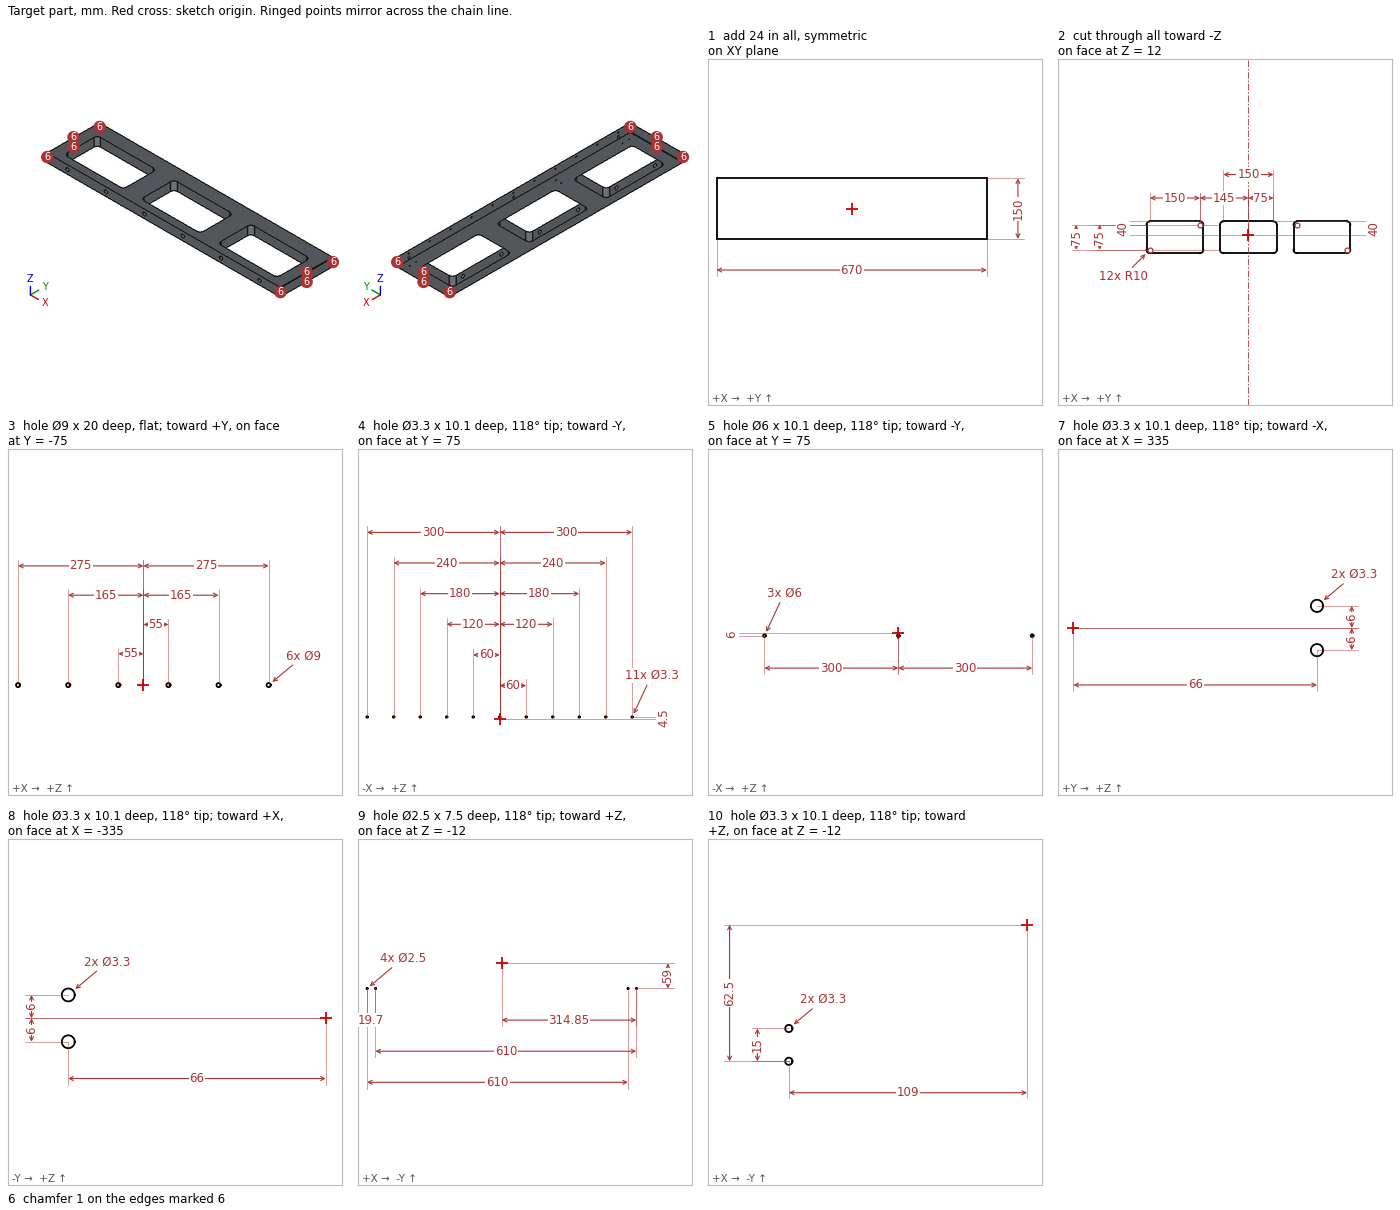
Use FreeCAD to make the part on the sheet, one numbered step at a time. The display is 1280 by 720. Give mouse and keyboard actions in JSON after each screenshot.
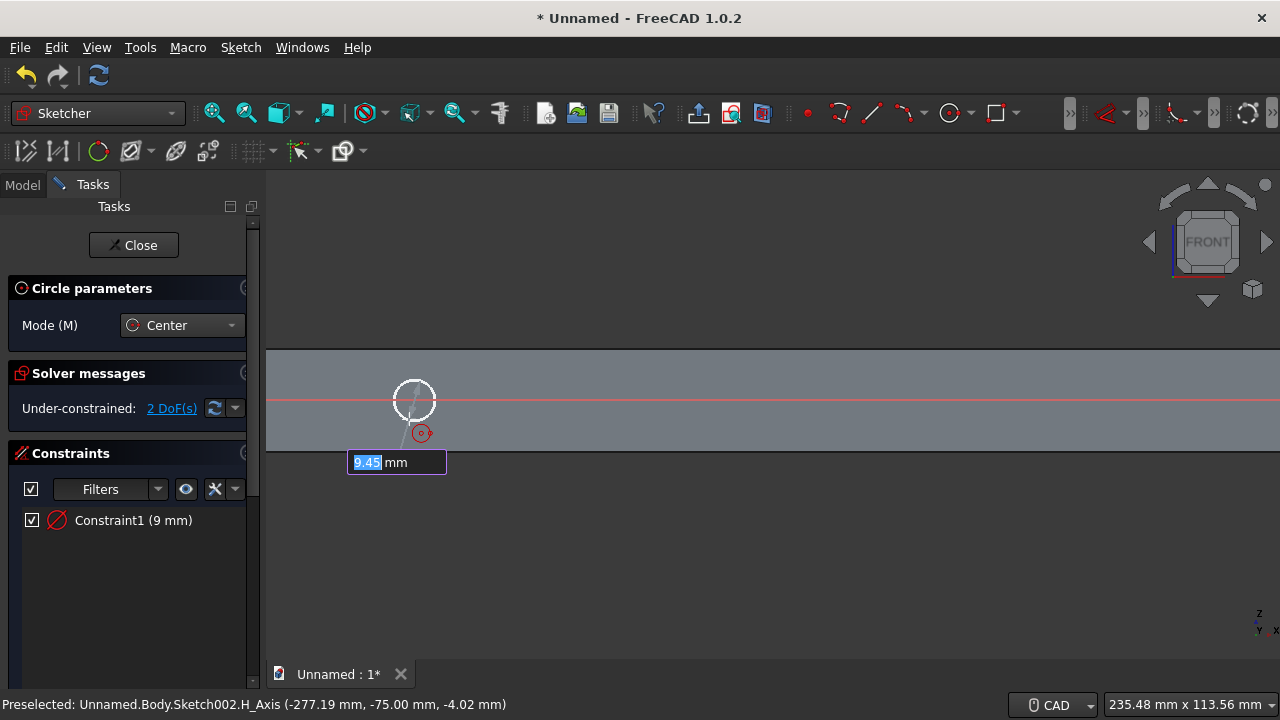
{"action": "type", "text": "9"}
{"action": "key", "text": "Return"}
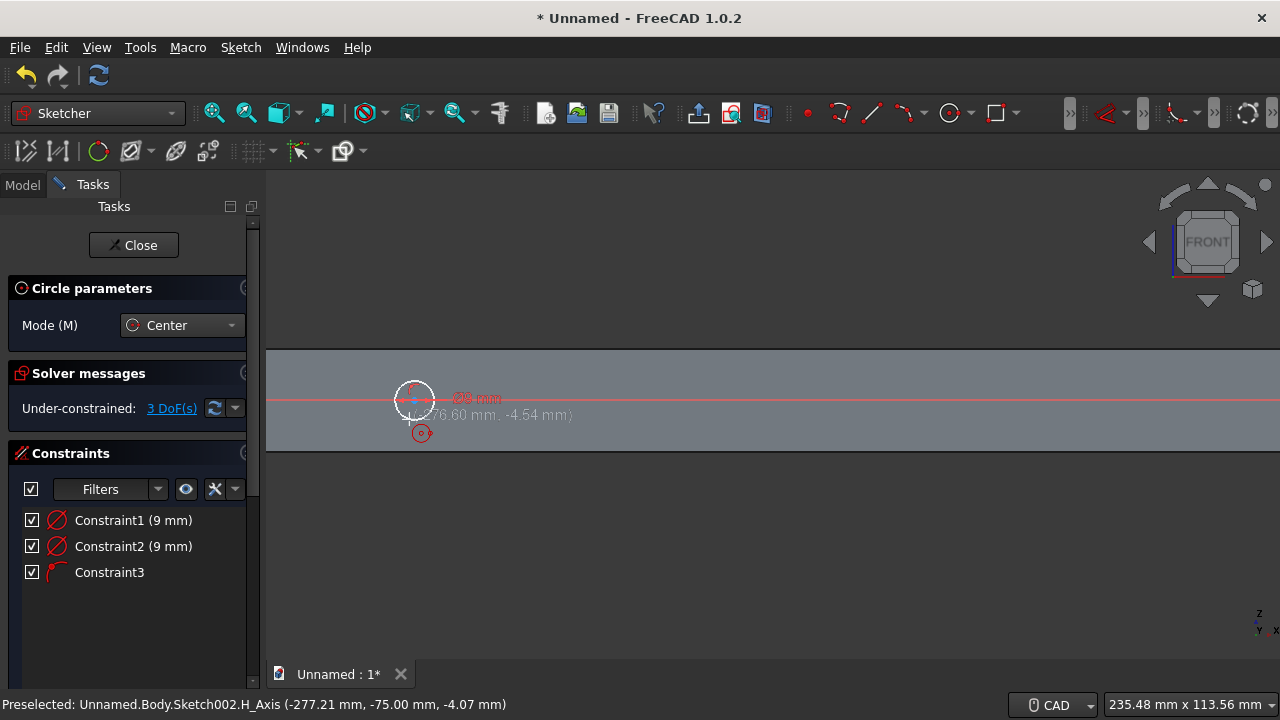
{"action": "scroll", "coordinate": [411, 419], "scroll_direction": "down", "scroll_amount": 7}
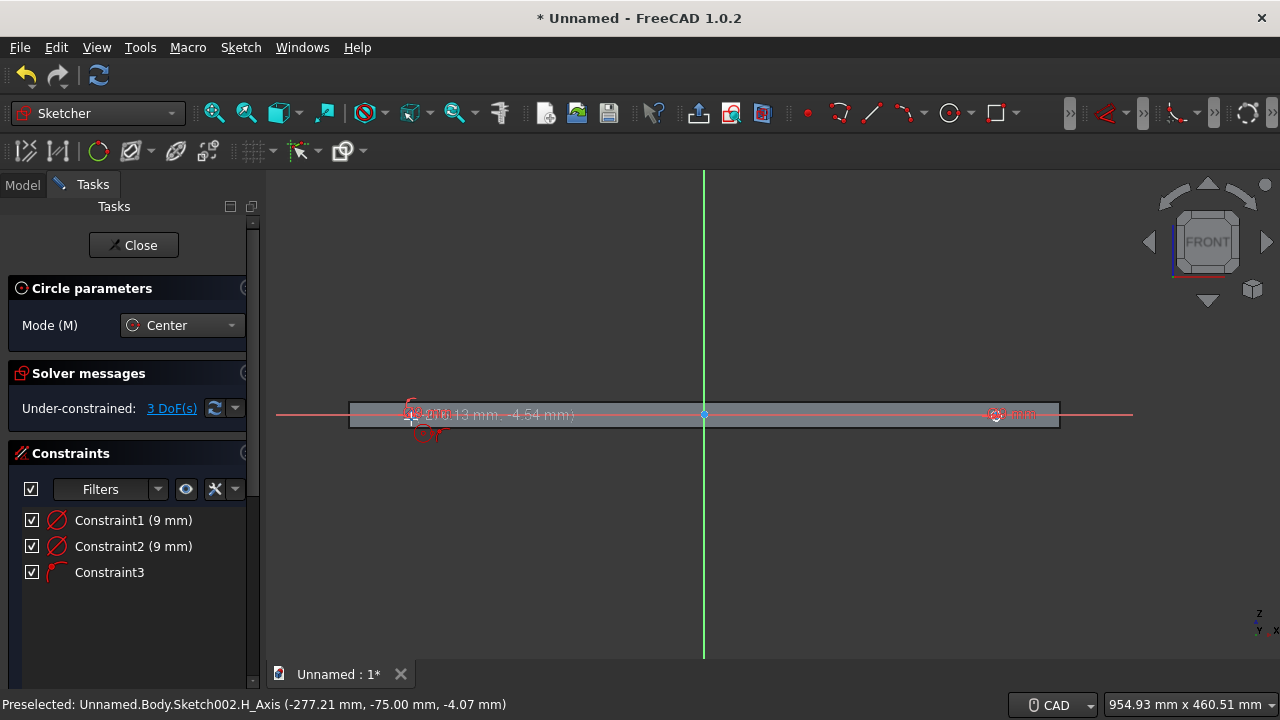
{"action": "left_click", "coordinate": [529, 415]}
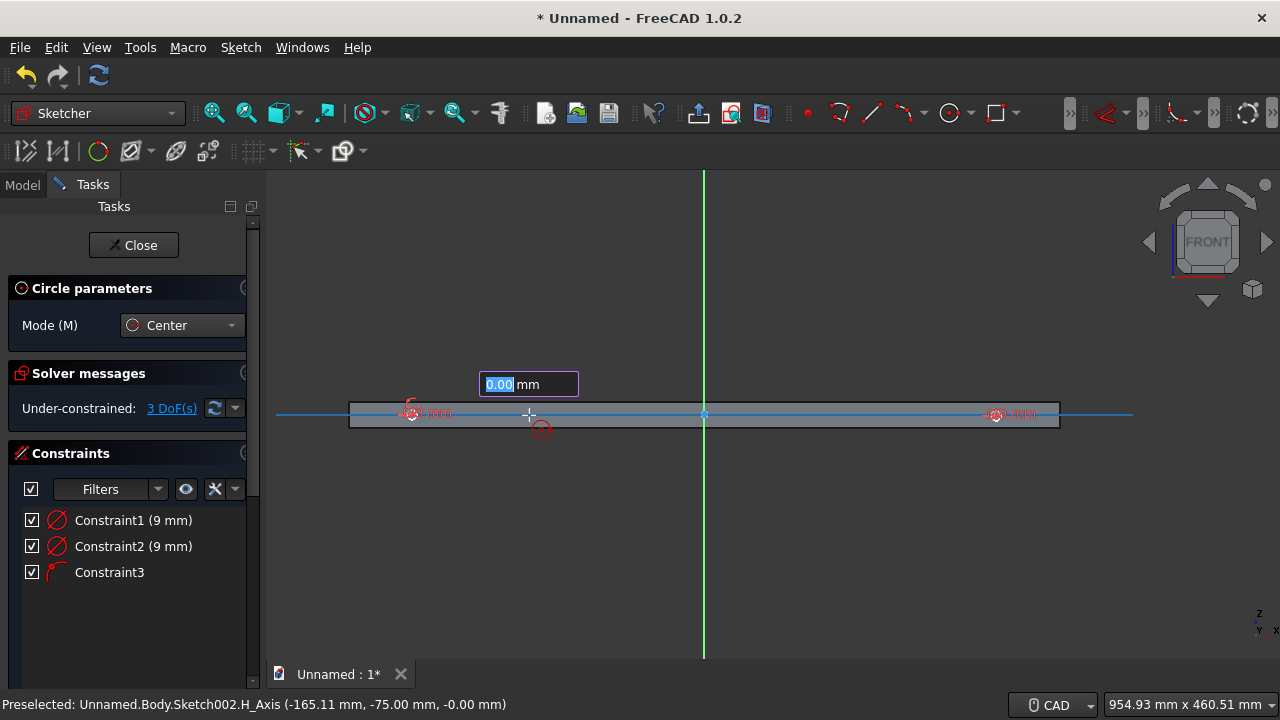
{"action": "scroll", "coordinate": [527, 419], "scroll_direction": "up", "scroll_amount": 7}
{"action": "mouse_move", "coordinate": [528, 419]}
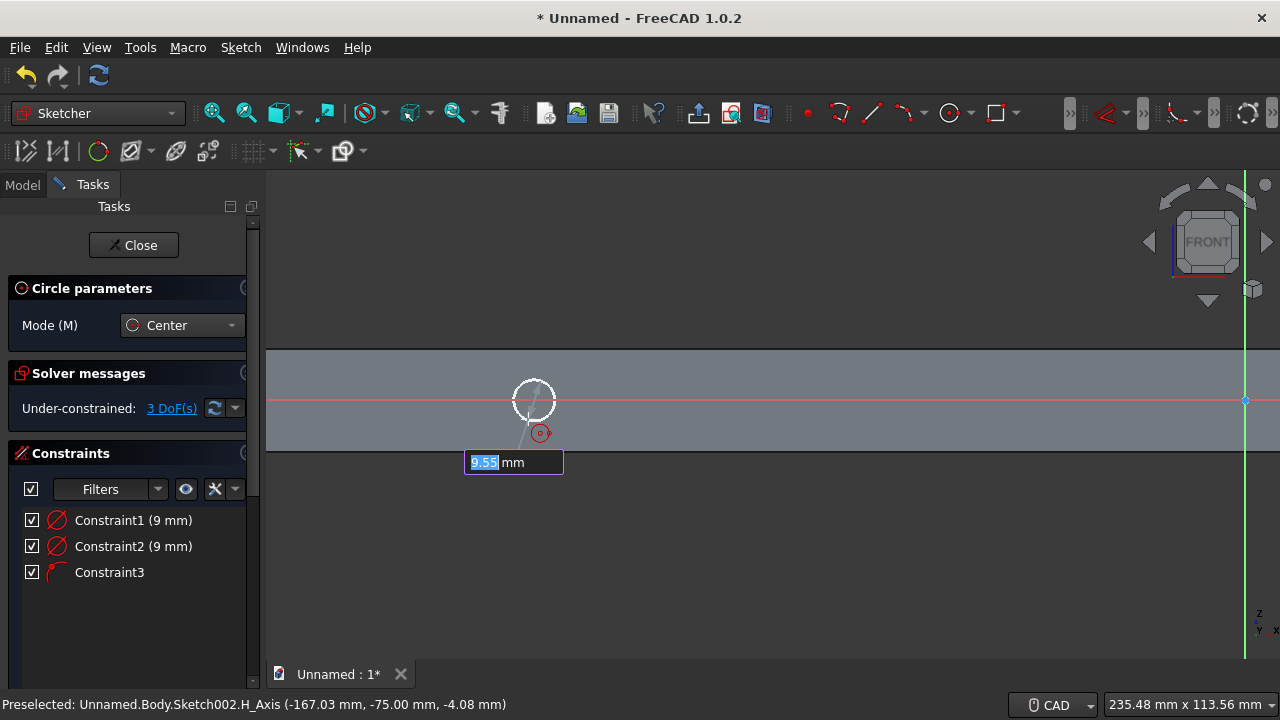
{"action": "type", "text": "9"}
{"action": "key", "text": "Return"}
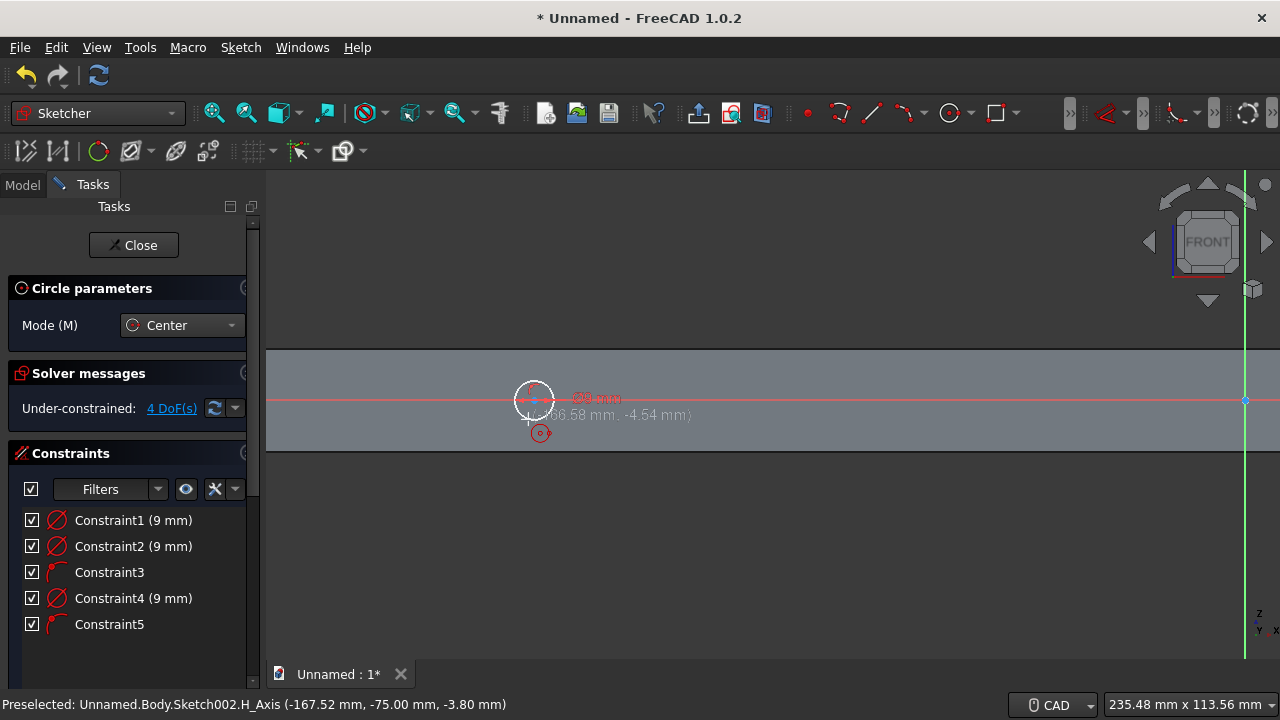
{"action": "scroll", "coordinate": [527, 419], "scroll_direction": "down", "scroll_amount": 7}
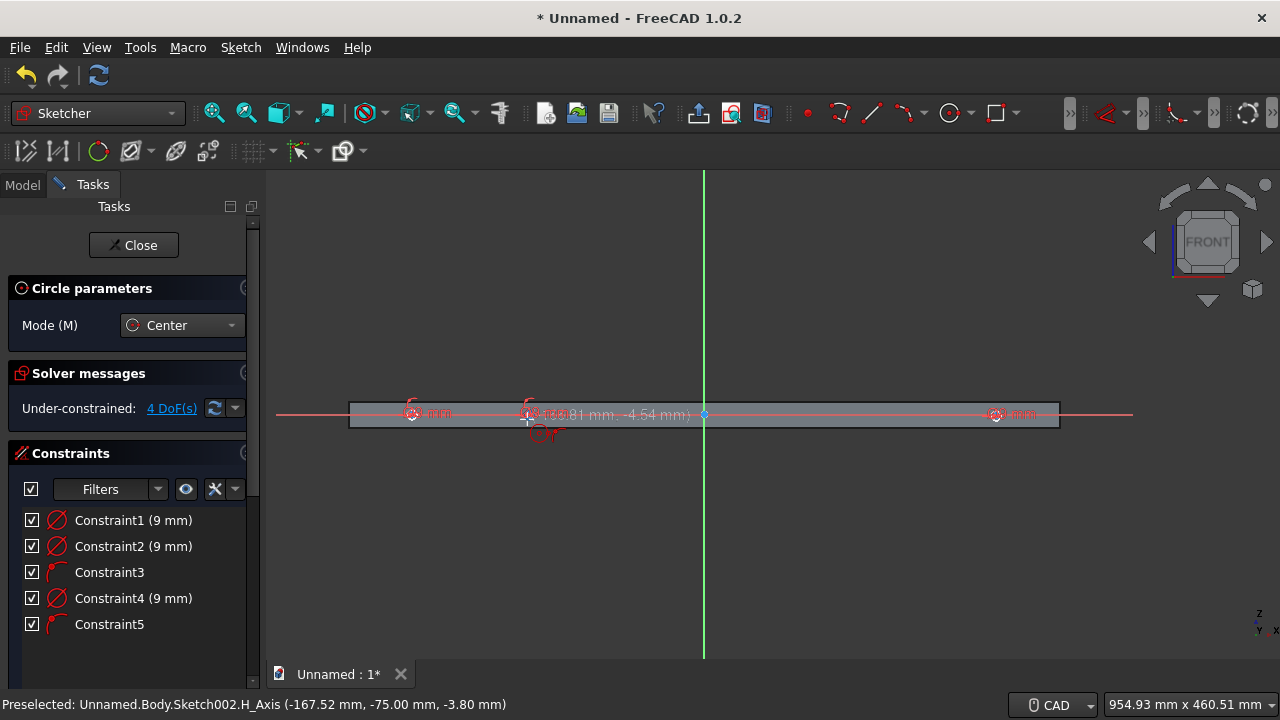
{"action": "left_click", "coordinate": [646, 415]}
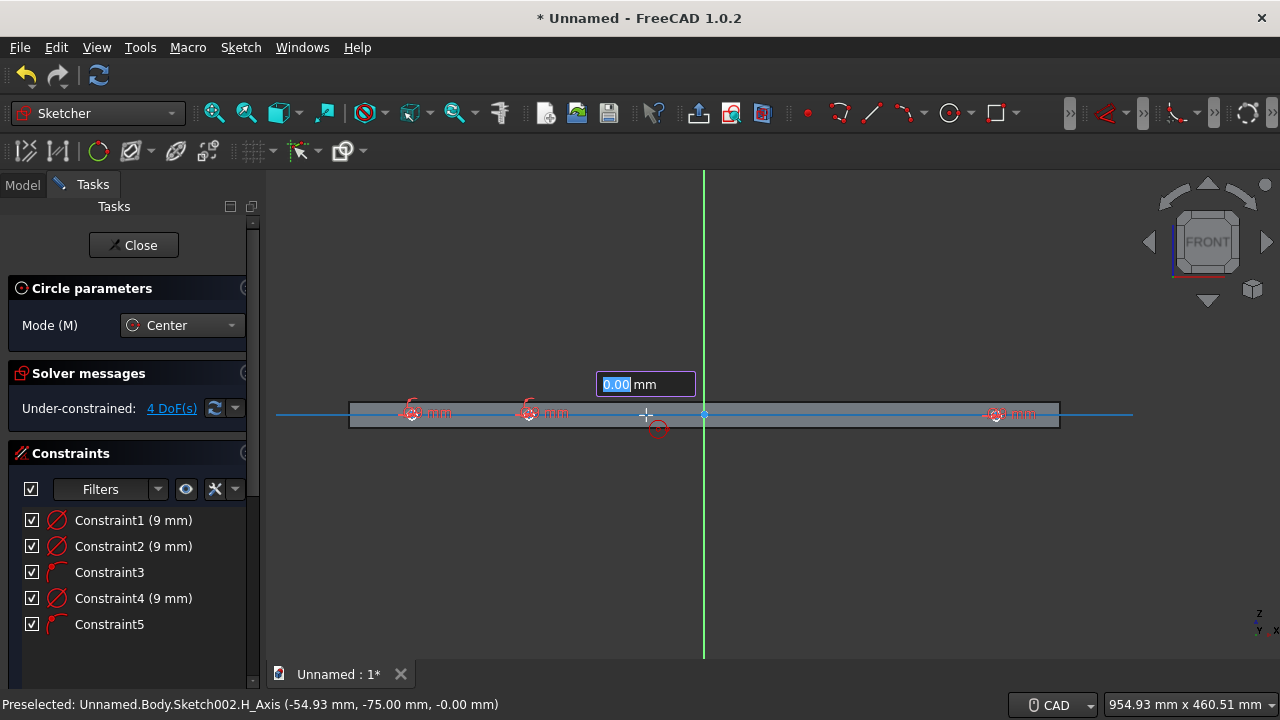
{"action": "scroll", "coordinate": [644, 419], "scroll_direction": "up", "scroll_amount": 7}
{"action": "mouse_move", "coordinate": [644, 419]}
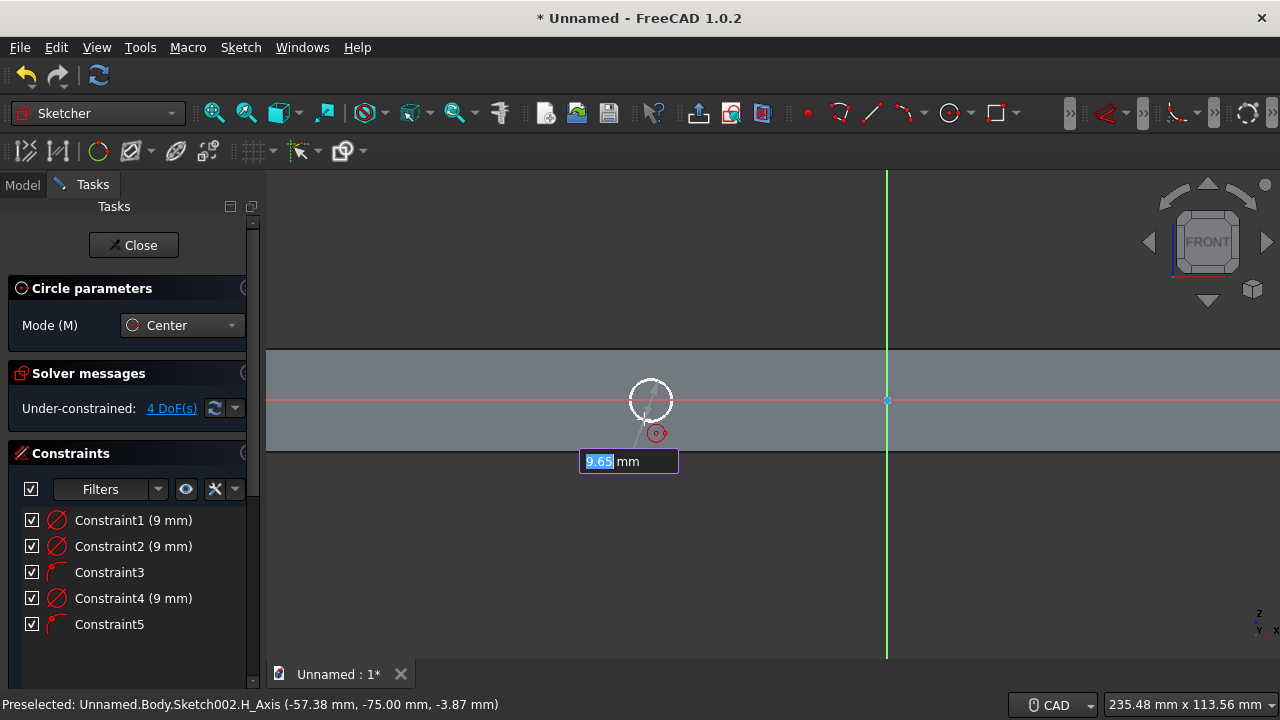
{"action": "type", "text": "9"}
{"action": "key", "text": "Return"}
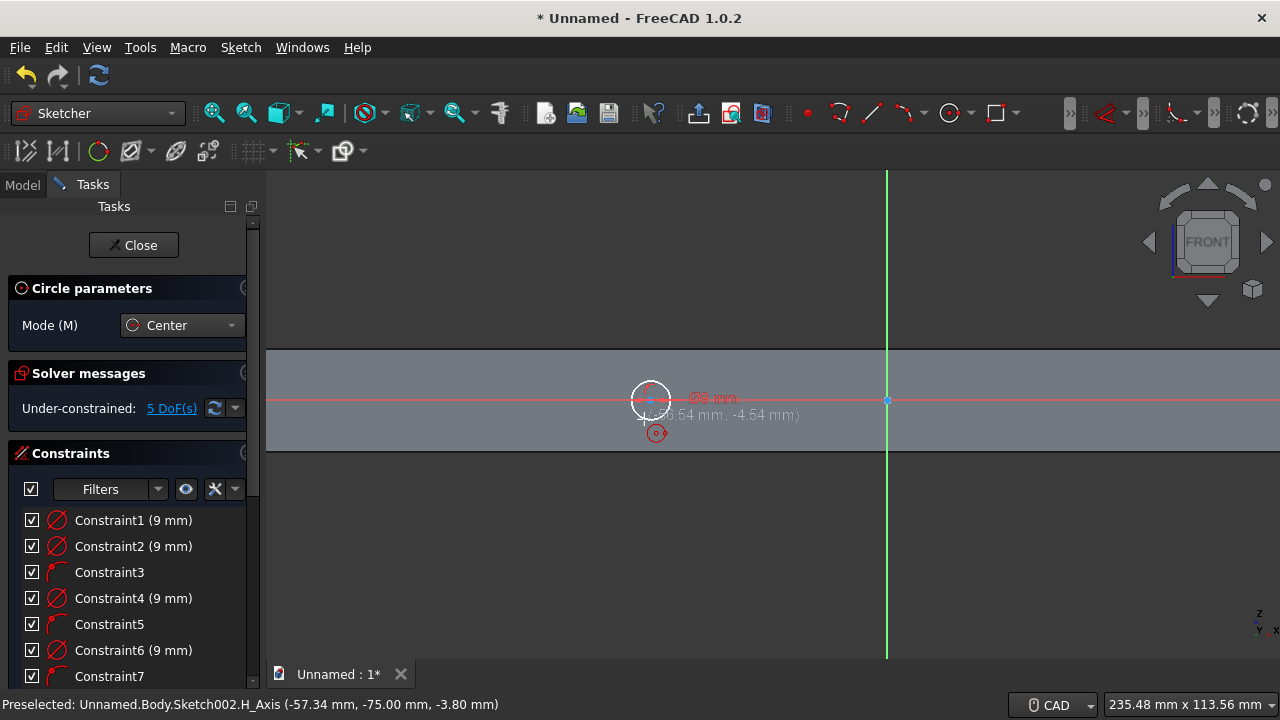
{"action": "scroll", "coordinate": [645, 419], "scroll_direction": "down", "scroll_amount": 7}